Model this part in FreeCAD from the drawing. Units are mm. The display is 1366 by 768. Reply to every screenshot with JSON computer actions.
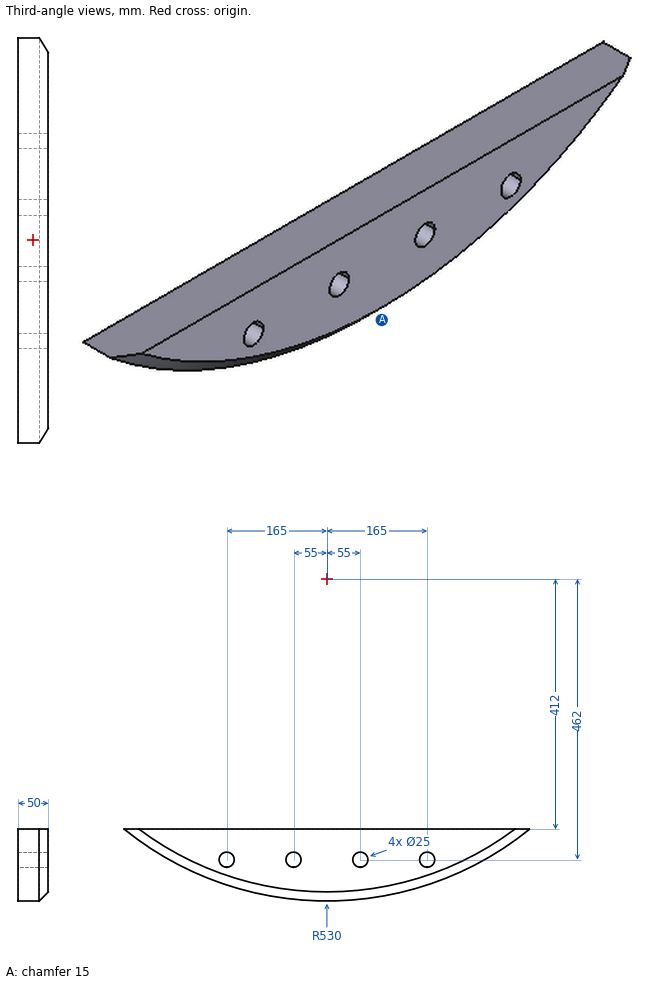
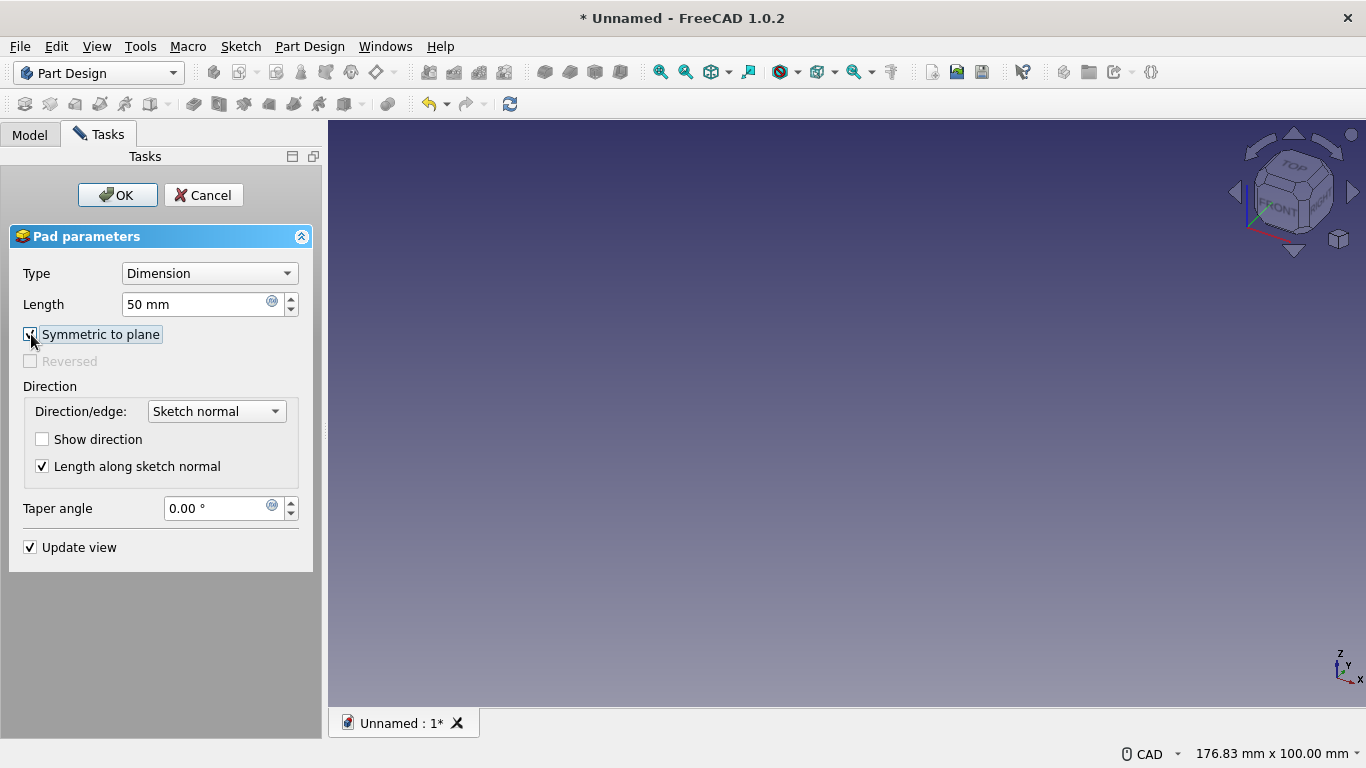
{"action": "left_click", "coordinate": [118, 195]}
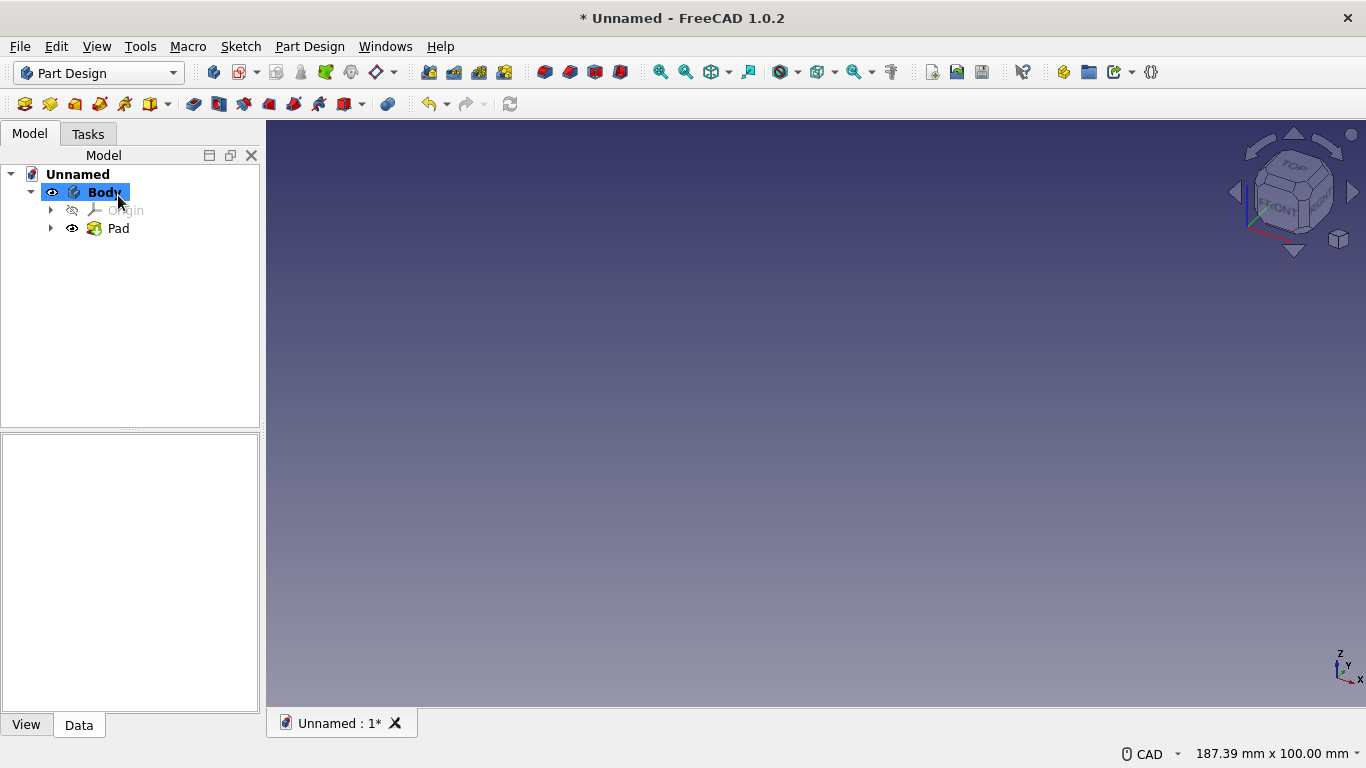
{"action": "left_click", "coordinate": [661, 72]}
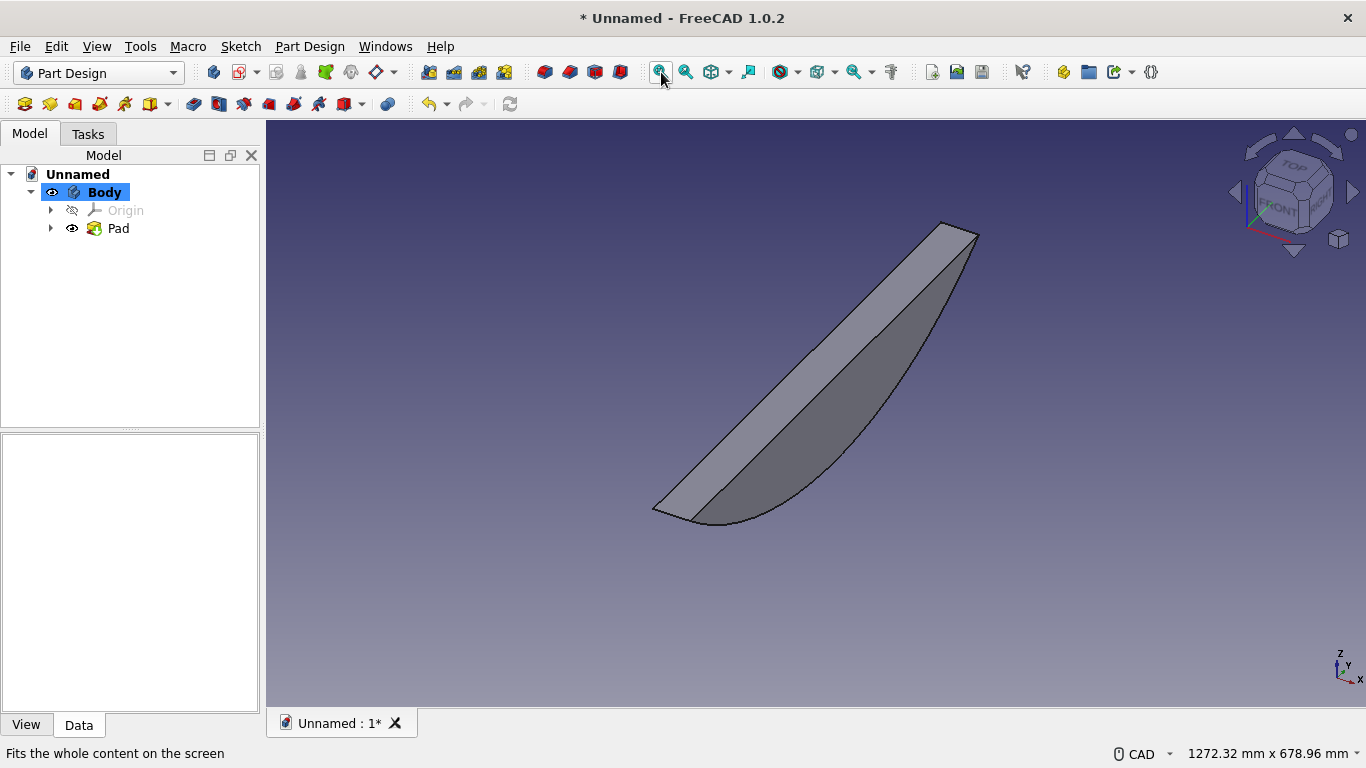
{"action": "left_click", "coordinate": [835, 419]}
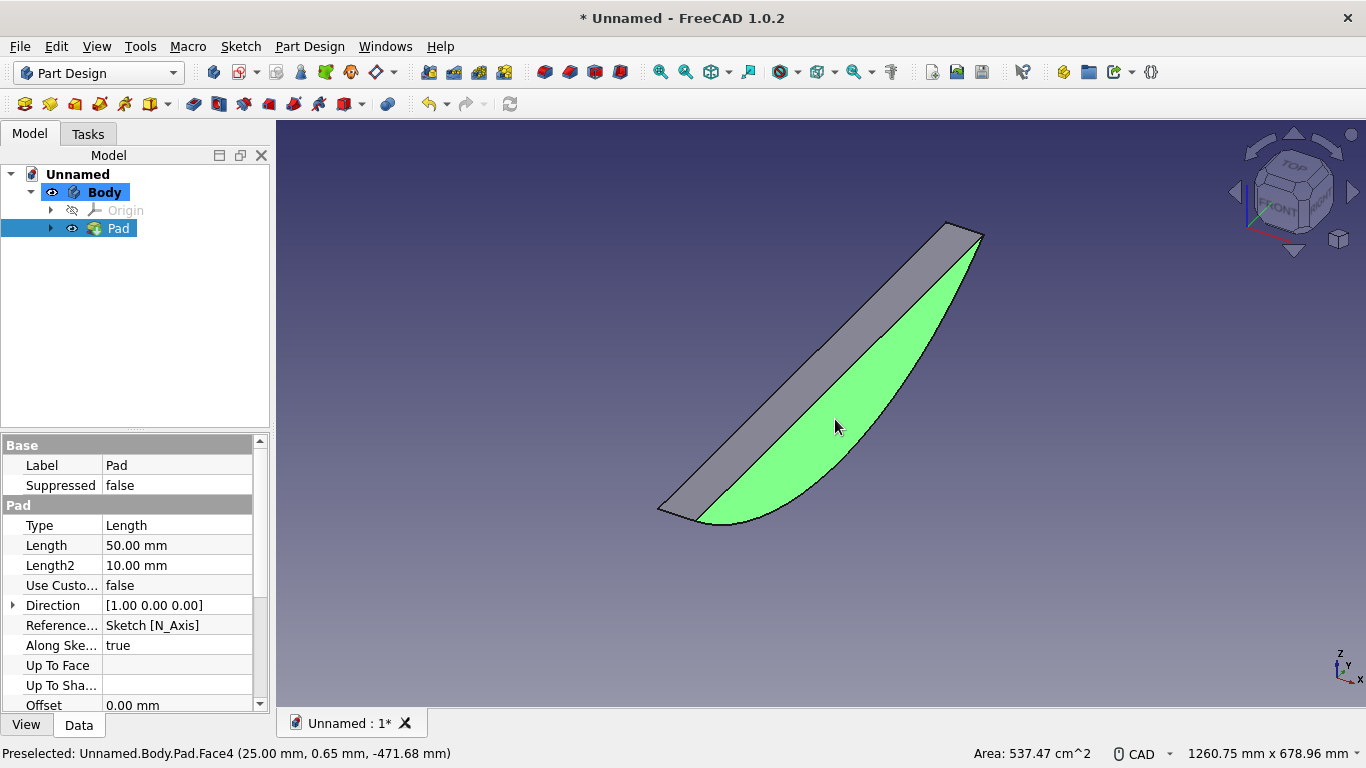
{"action": "left_click", "coordinate": [238, 72]}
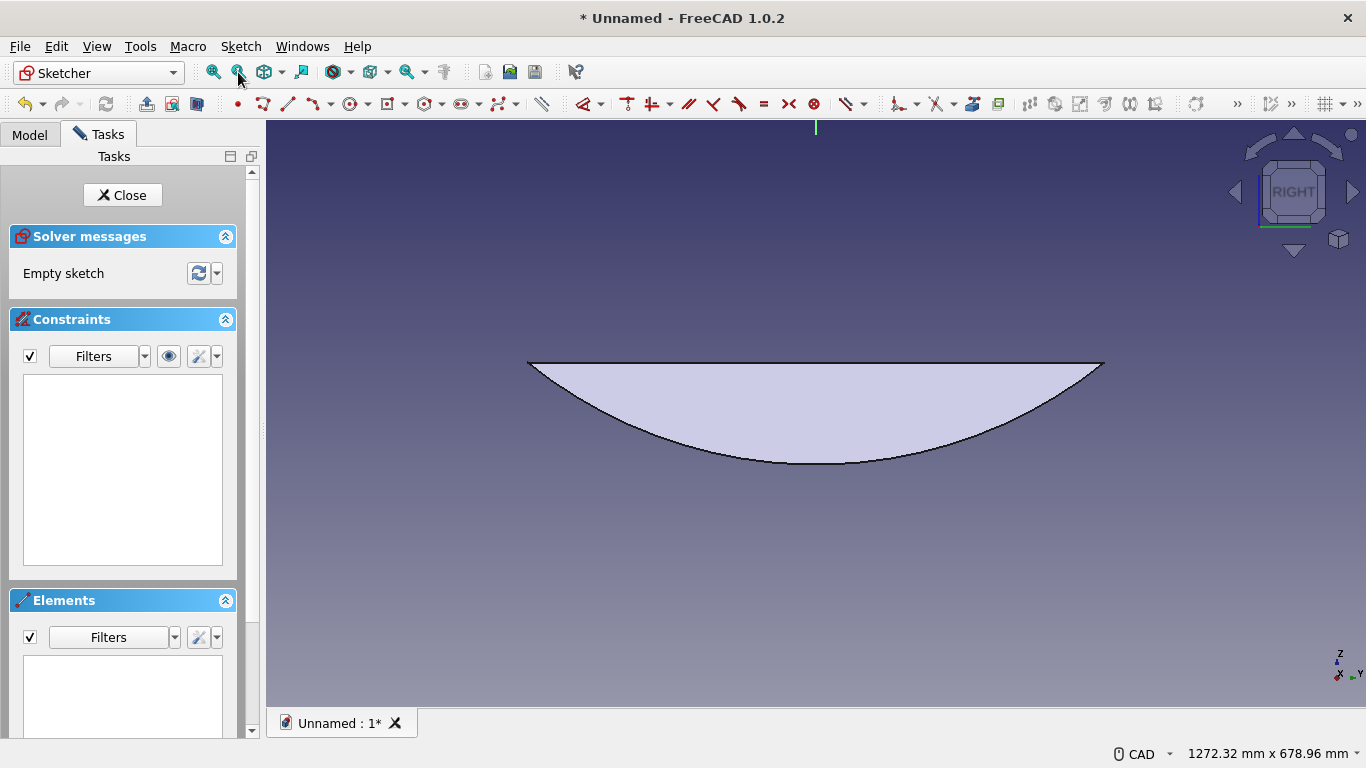
{"action": "scroll", "coordinate": [608, 679], "scroll_direction": "down", "scroll_amount": 2}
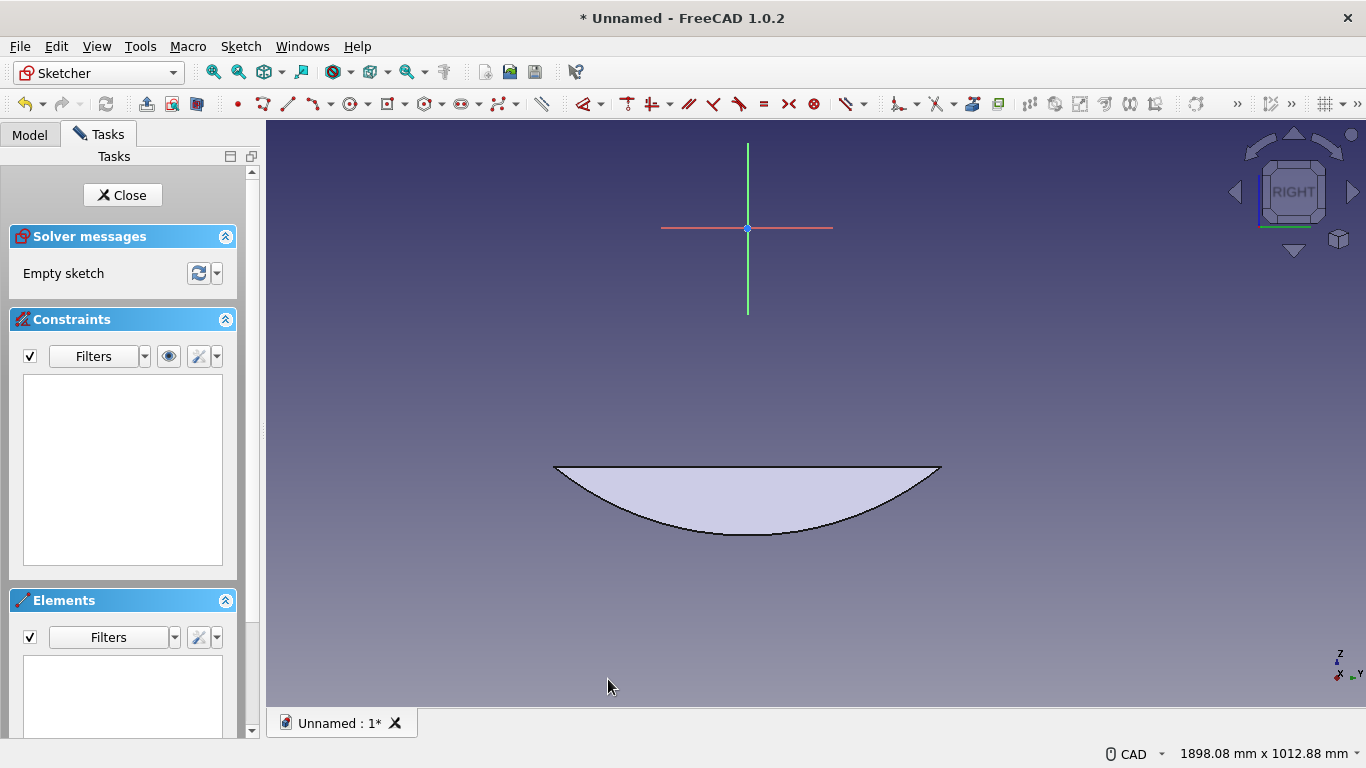
{"action": "scroll", "coordinate": [748, 269], "scroll_direction": "up", "scroll_amount": 2}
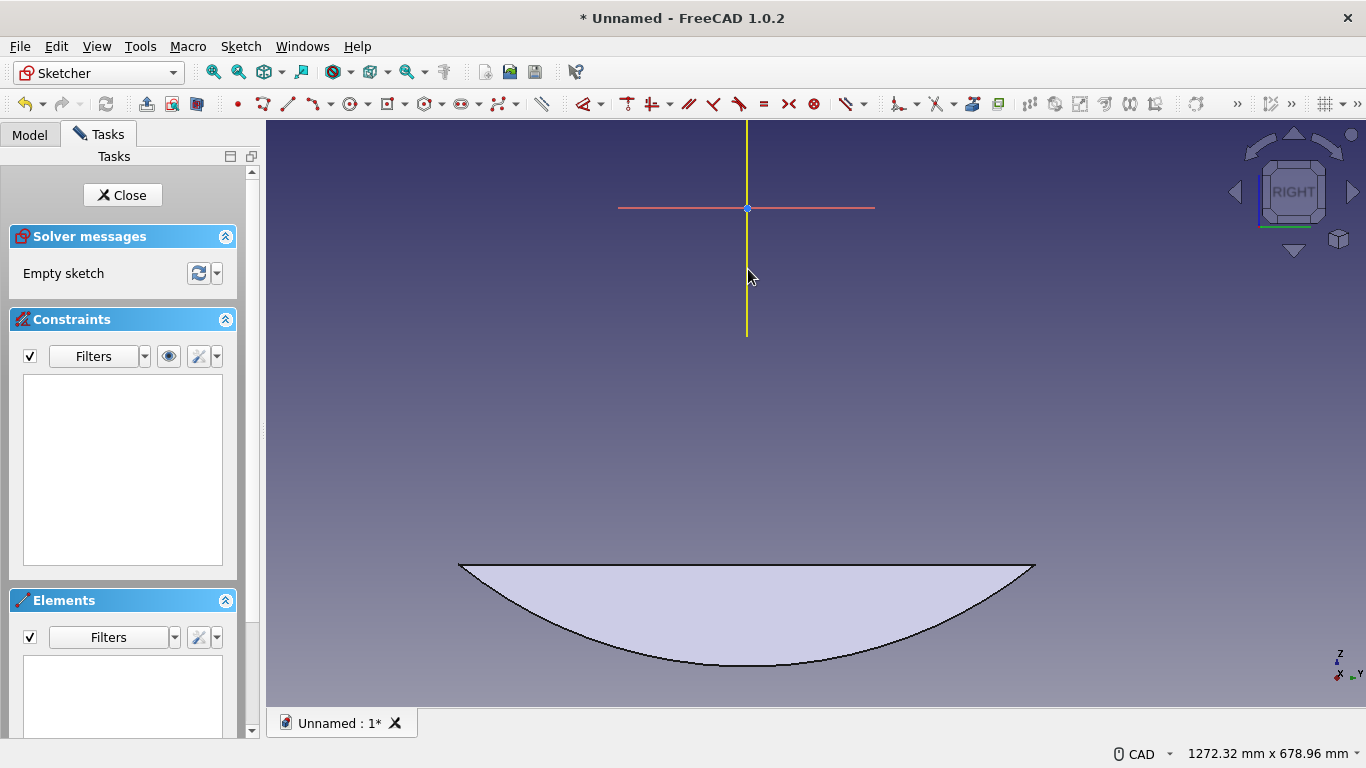
{"action": "left_click", "coordinate": [350, 104]}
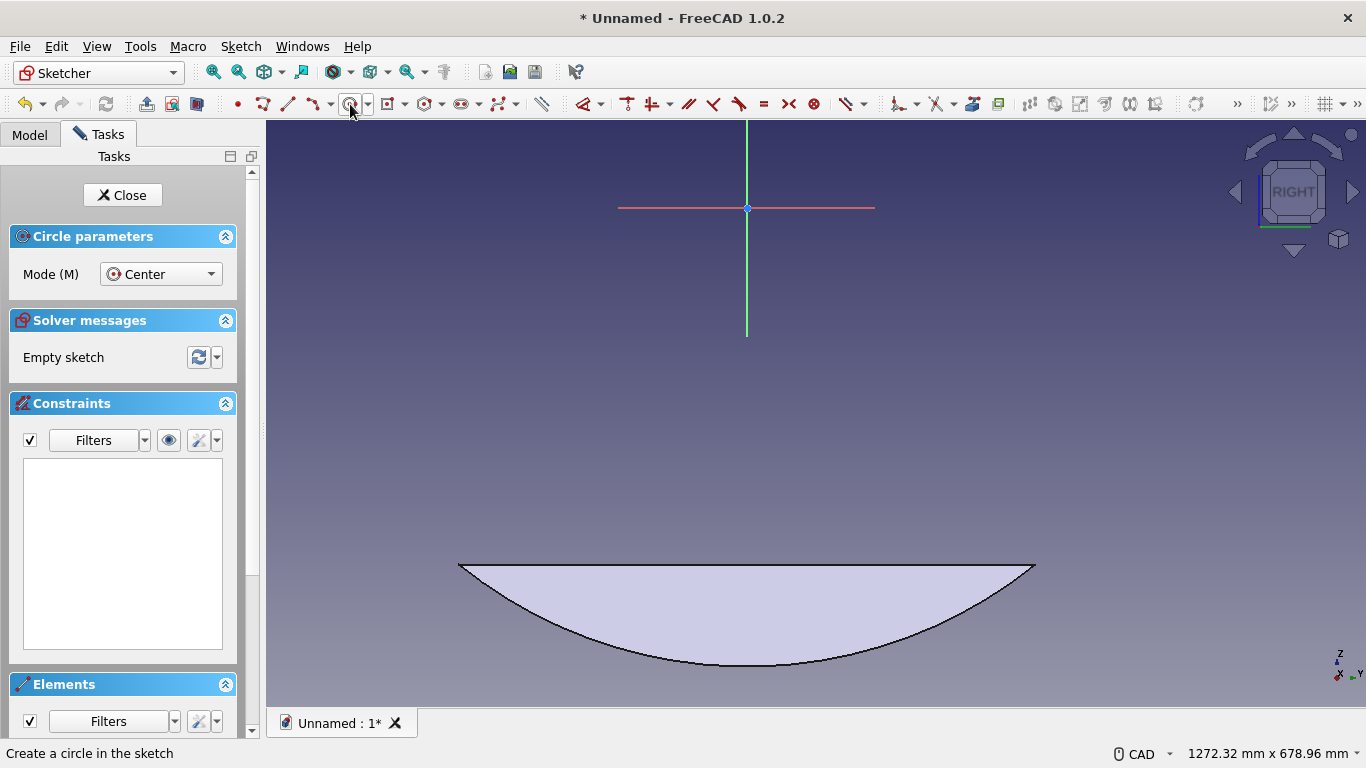
{"action": "scroll", "coordinate": [795, 608], "scroll_direction": "up", "scroll_amount": 4}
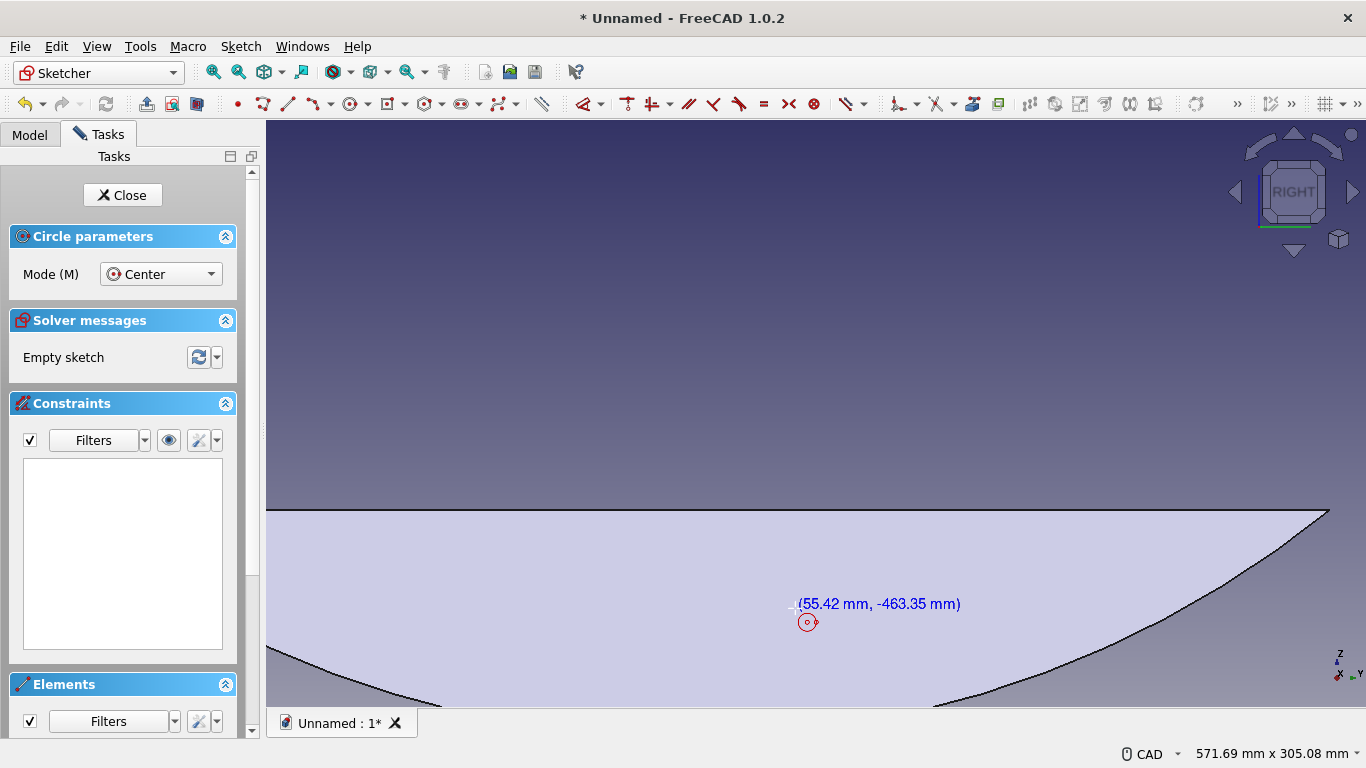
{"action": "left_click", "coordinate": [794, 607]}
{"action": "mouse_move", "coordinate": [811, 590]}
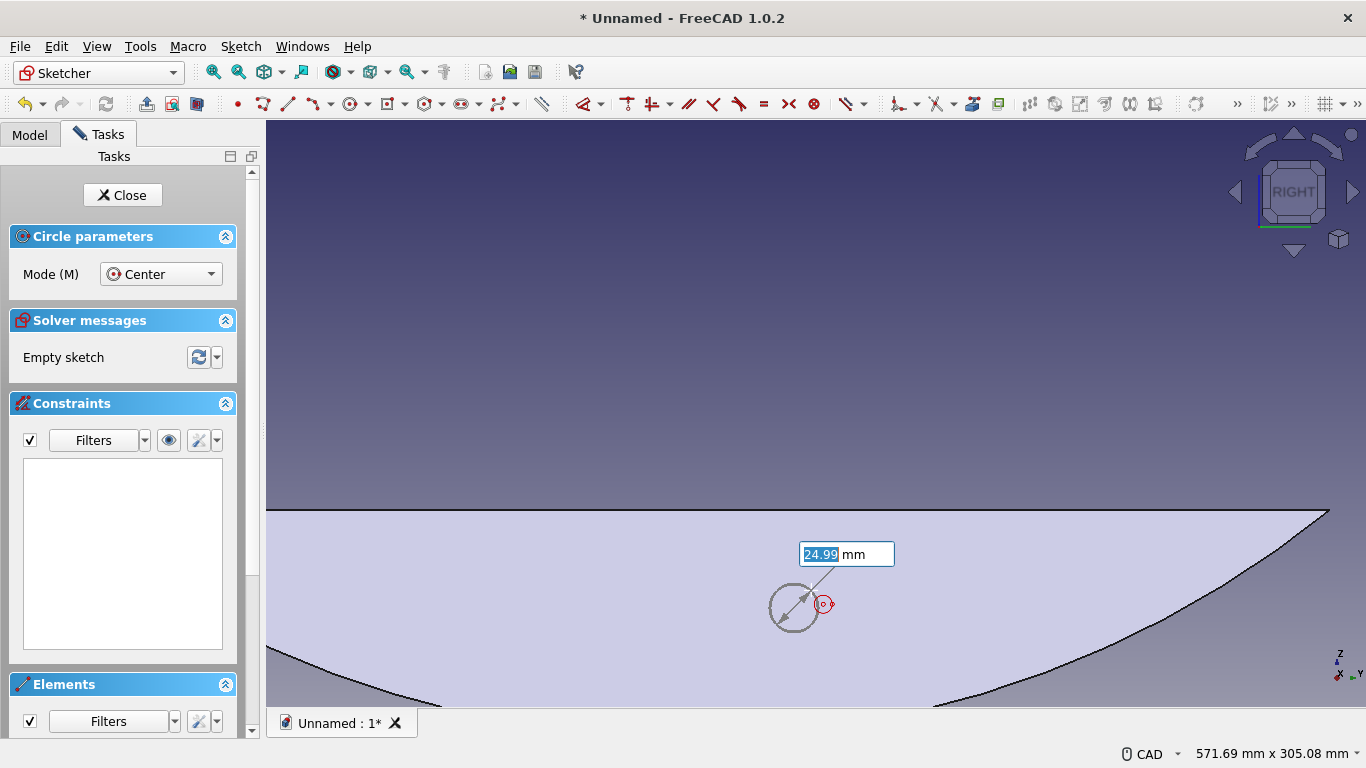
{"action": "type", "text": "25"}
{"action": "key", "text": "Return"}